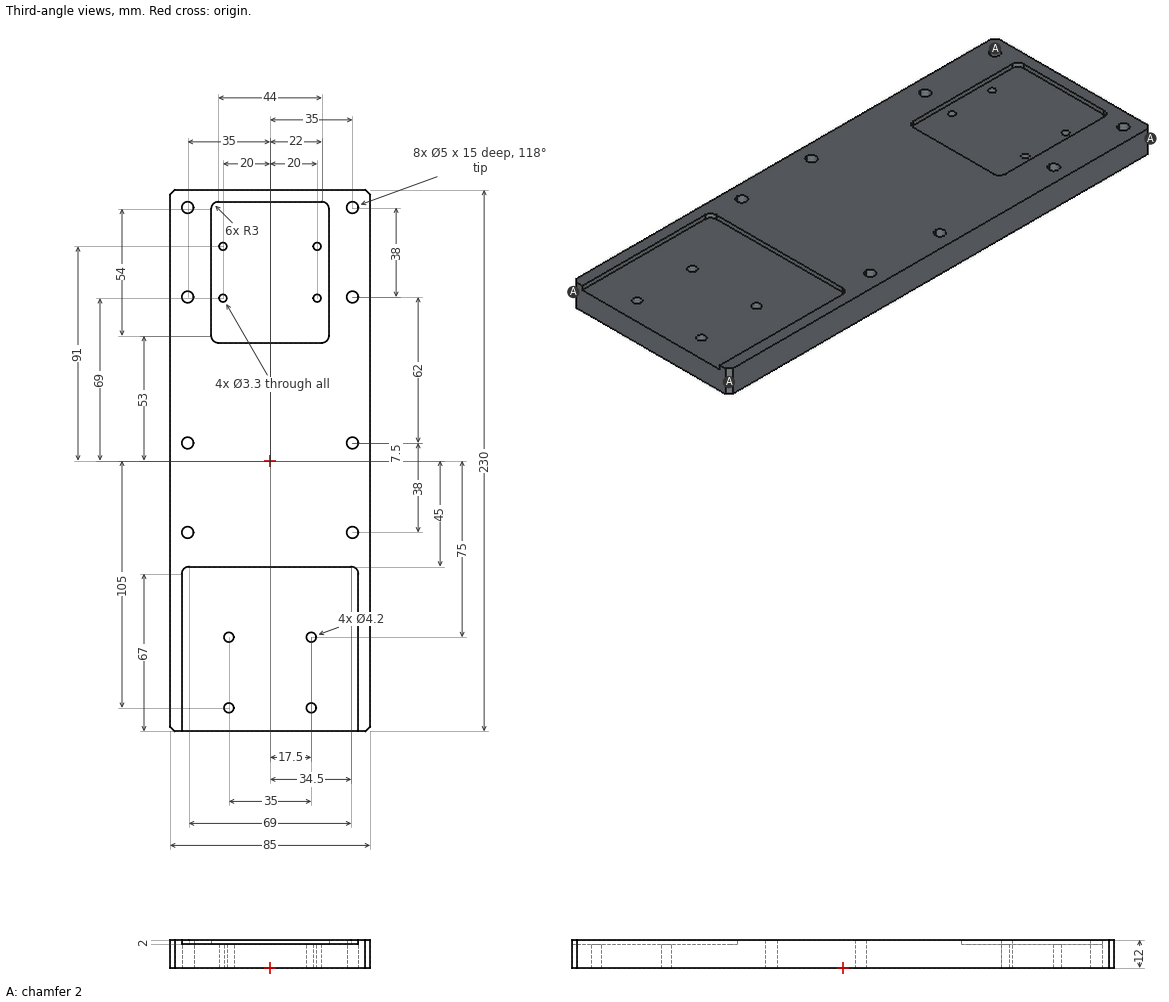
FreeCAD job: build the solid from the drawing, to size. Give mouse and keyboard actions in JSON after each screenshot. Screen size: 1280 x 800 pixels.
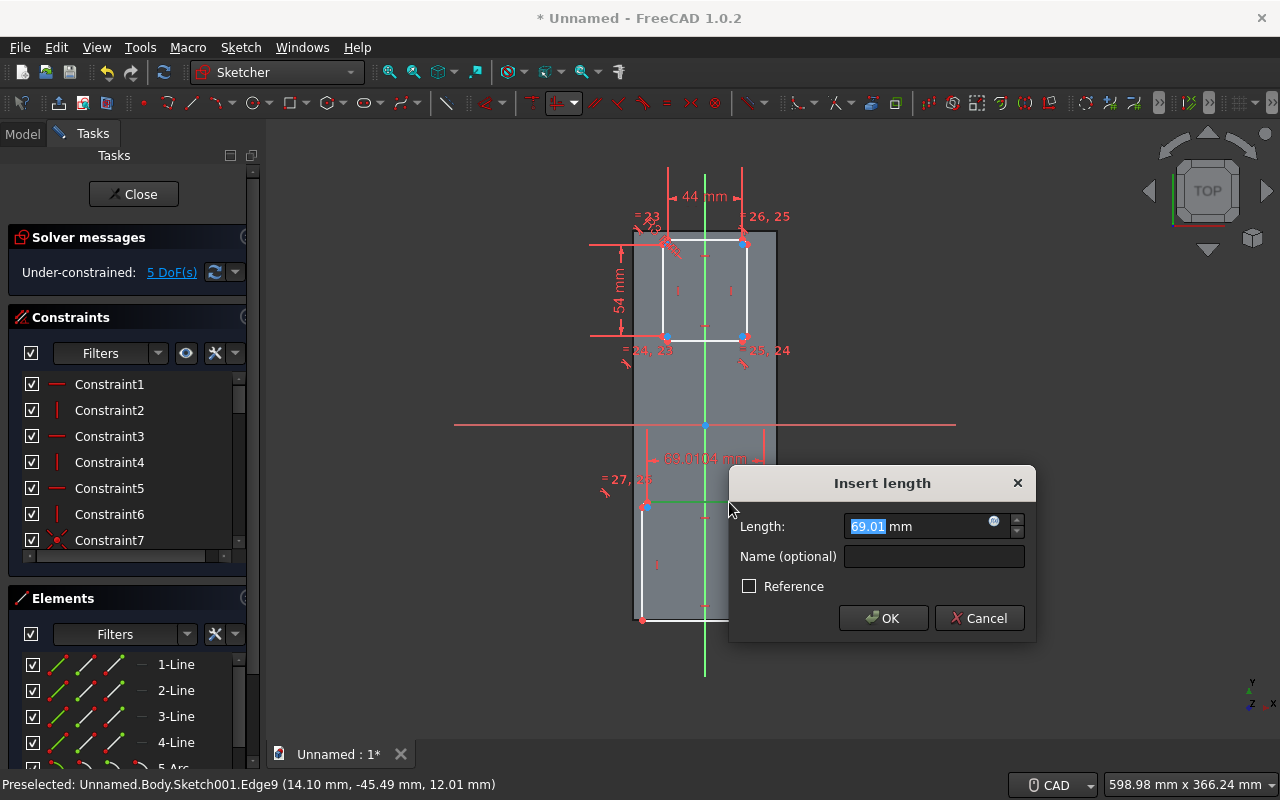
{"action": "type", "text": "69"}
{"action": "key", "text": "Return"}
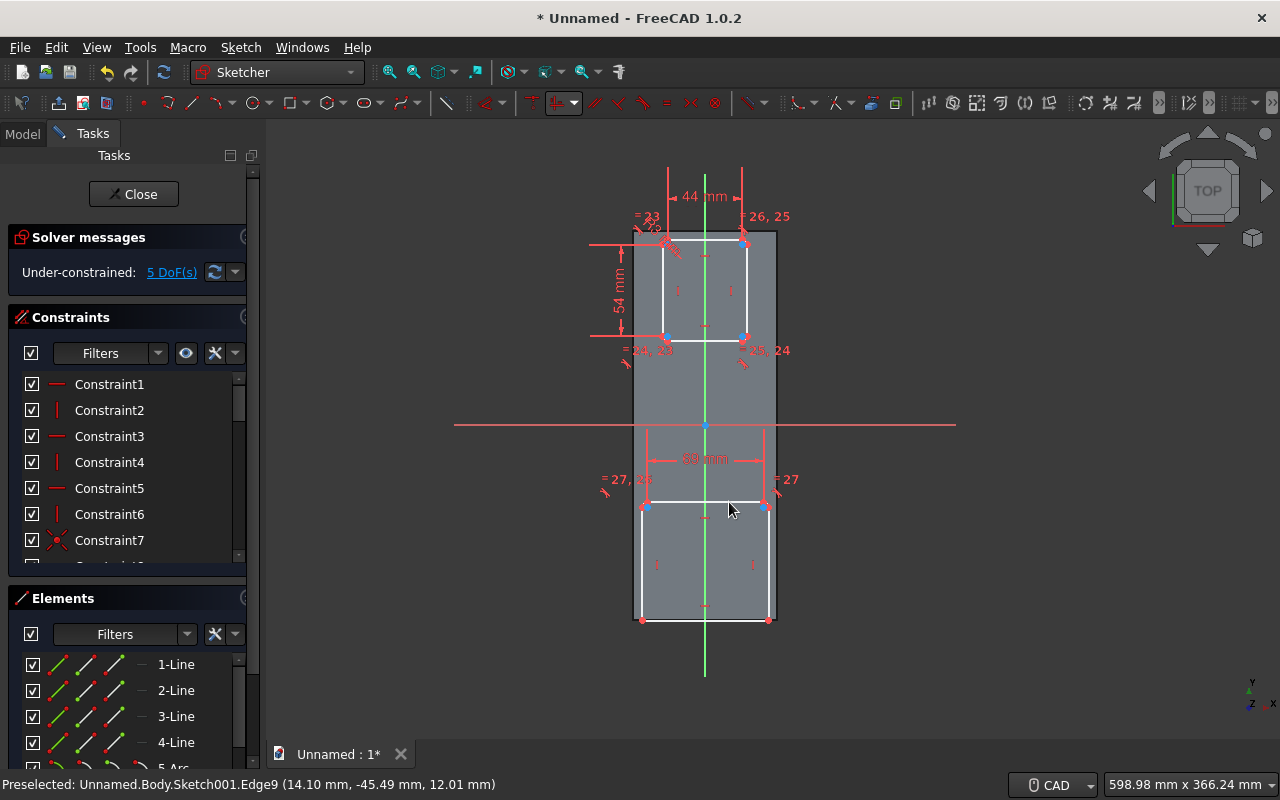
{"action": "left_click", "coordinate": [642, 541]}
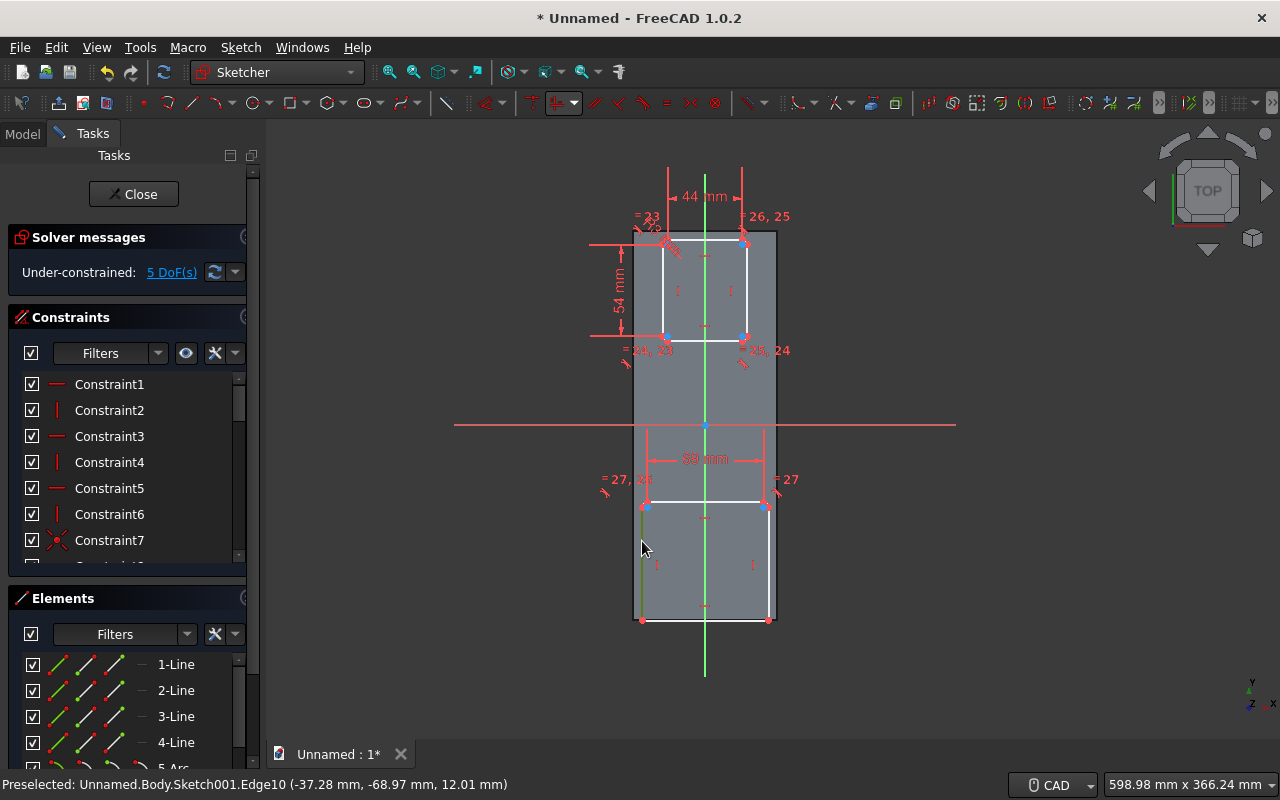
{"action": "key", "text": "i"}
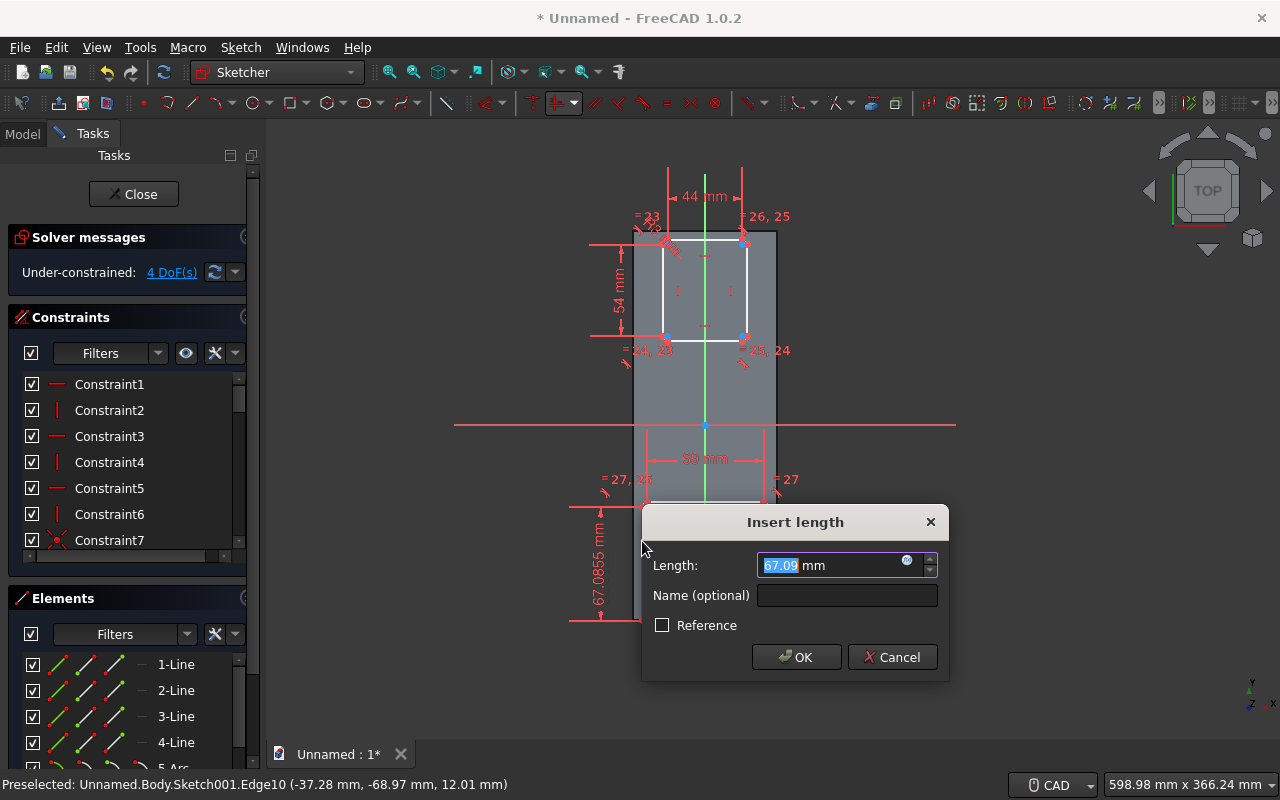
{"action": "type", "text": "67"}
{"action": "key", "text": "Return"}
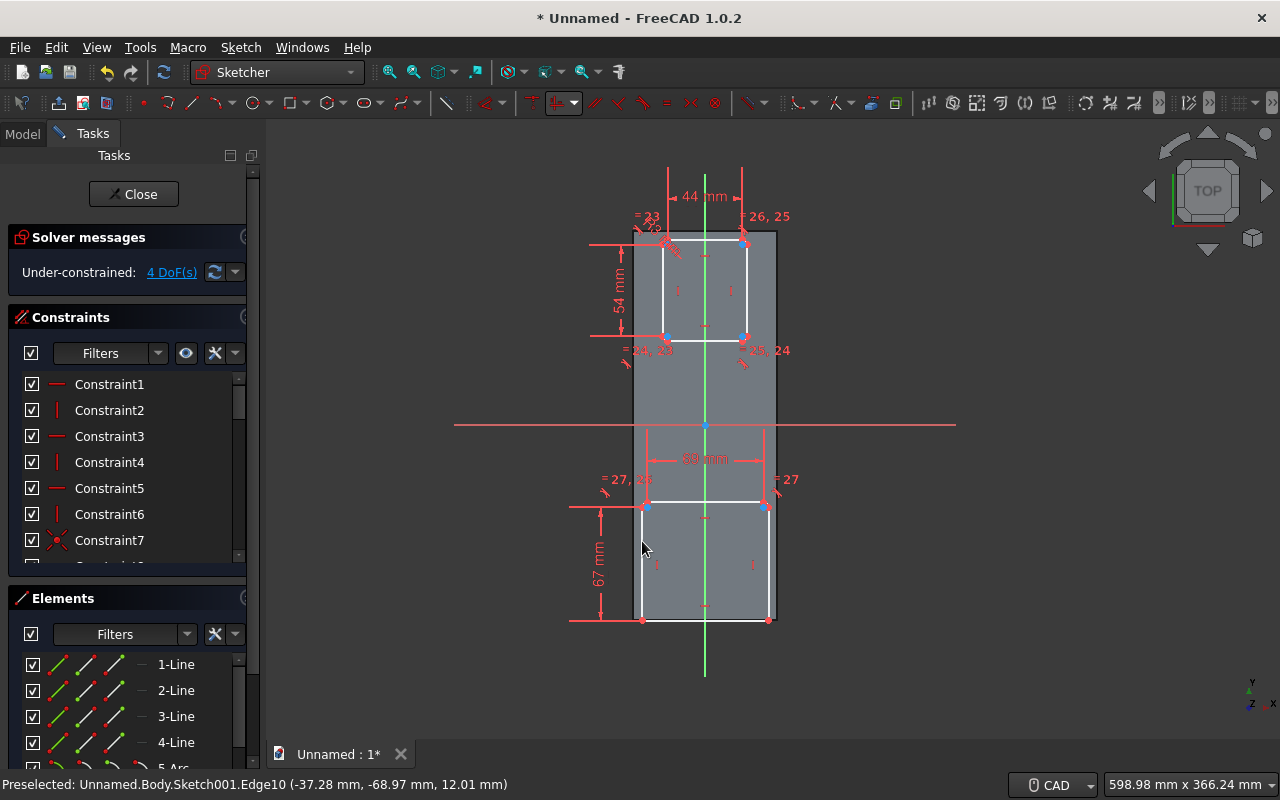
{"action": "scroll", "coordinate": [742, 240], "scroll_direction": "up", "scroll_amount": 5}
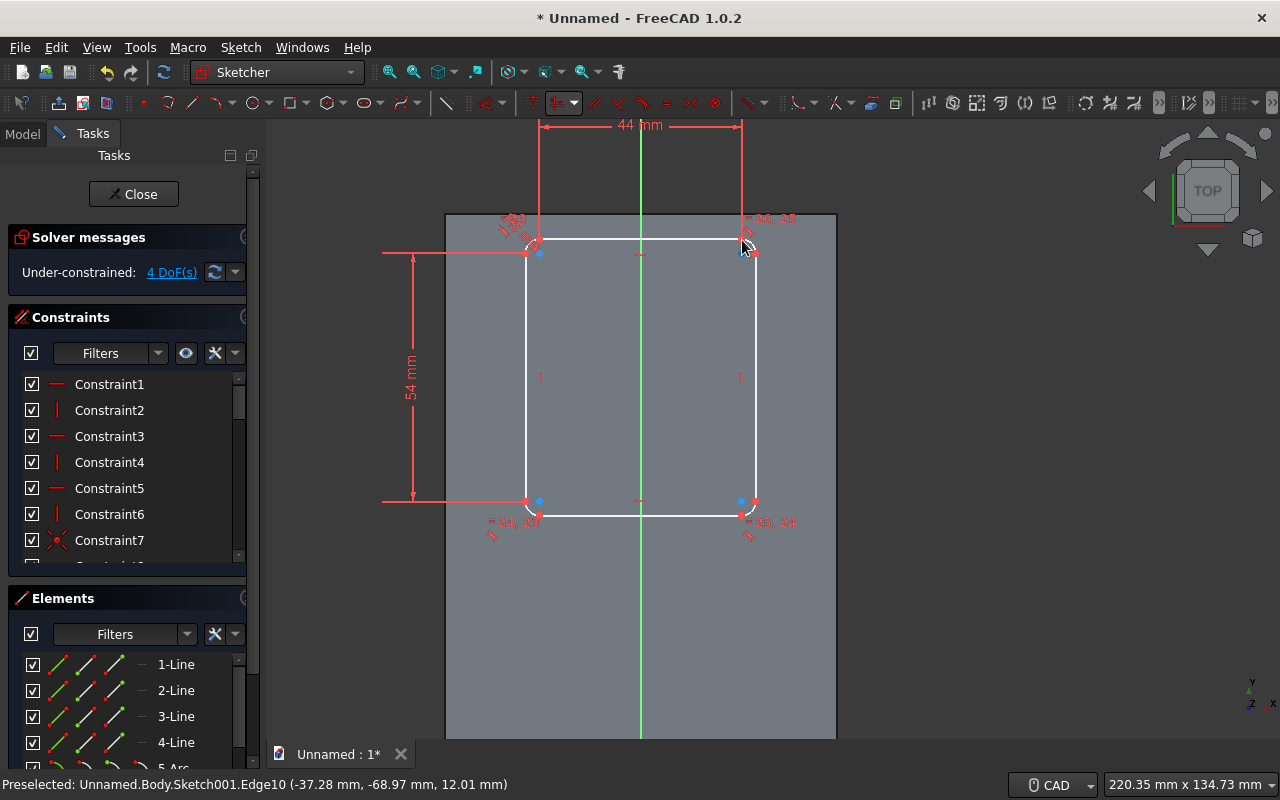
{"action": "left_click", "coordinate": [742, 239]}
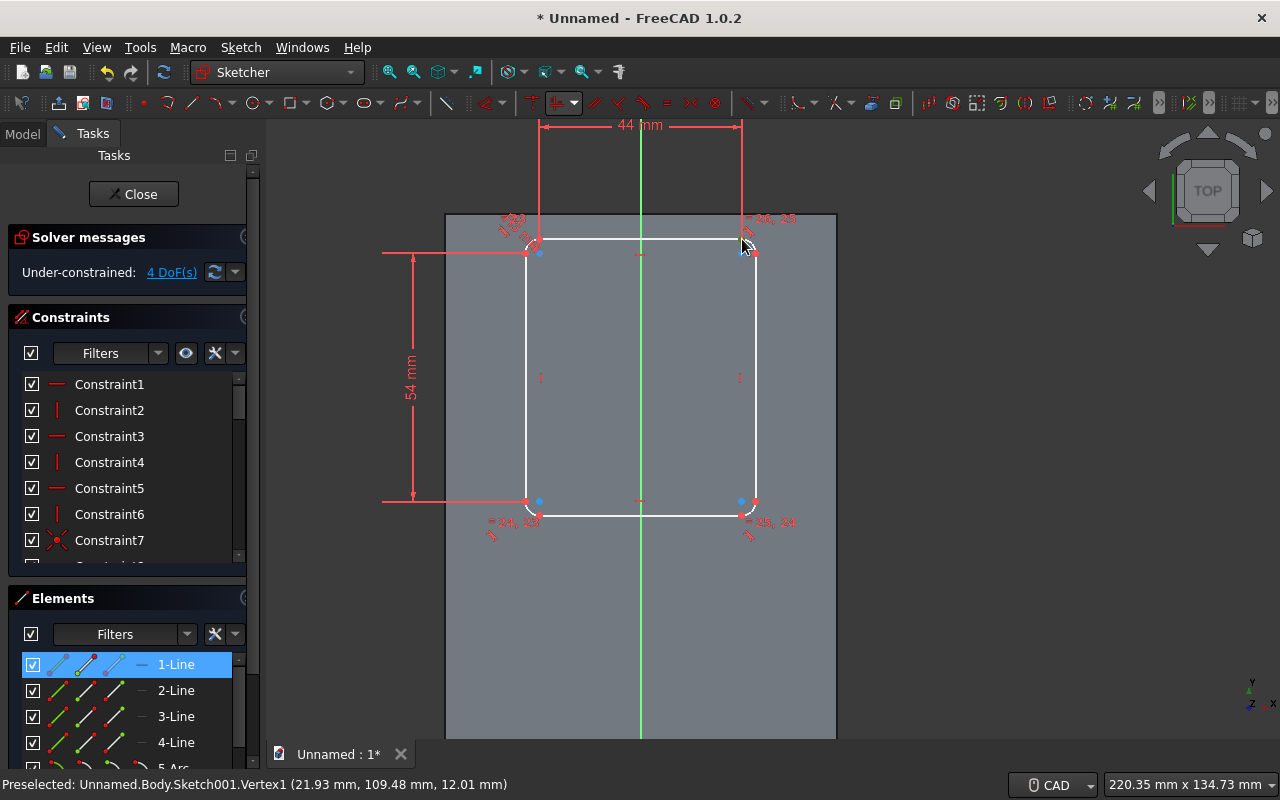
{"action": "key", "text": "l"}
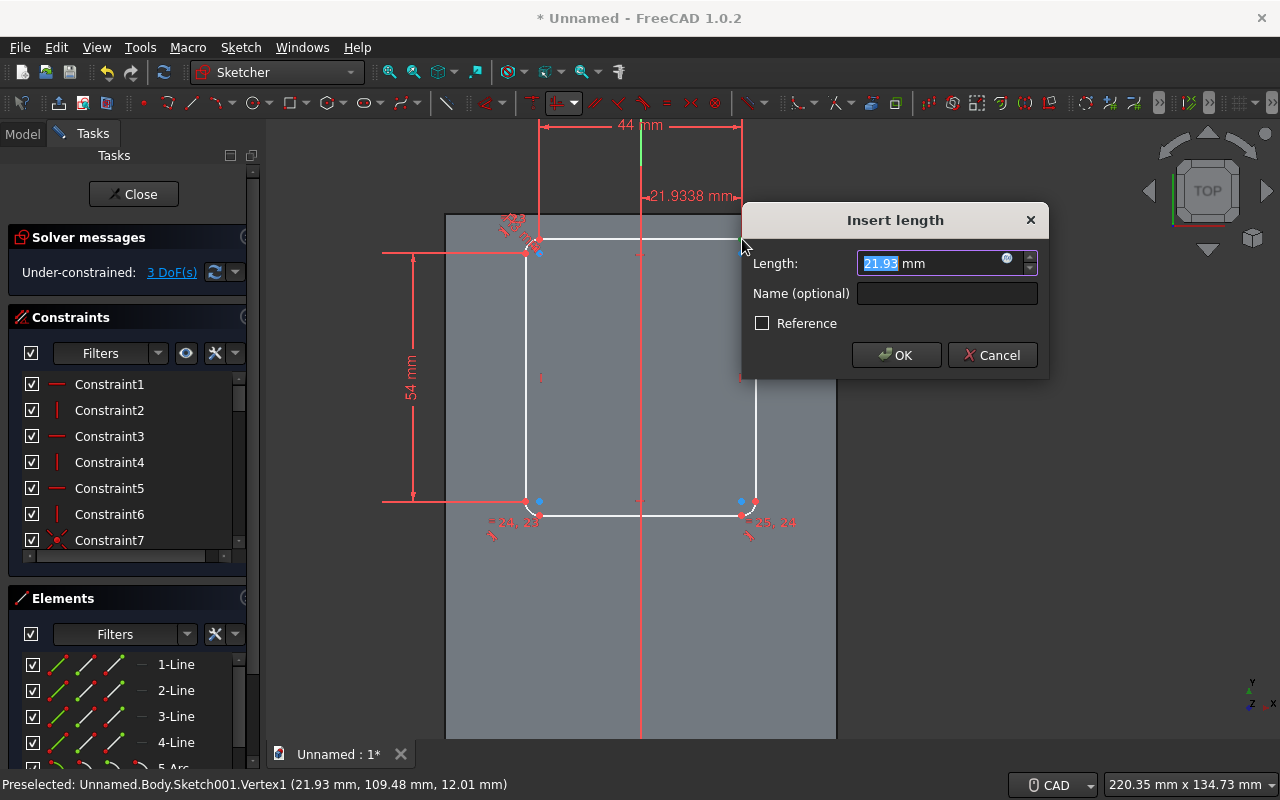
{"action": "type", "text": "22"}
{"action": "key", "text": "Return"}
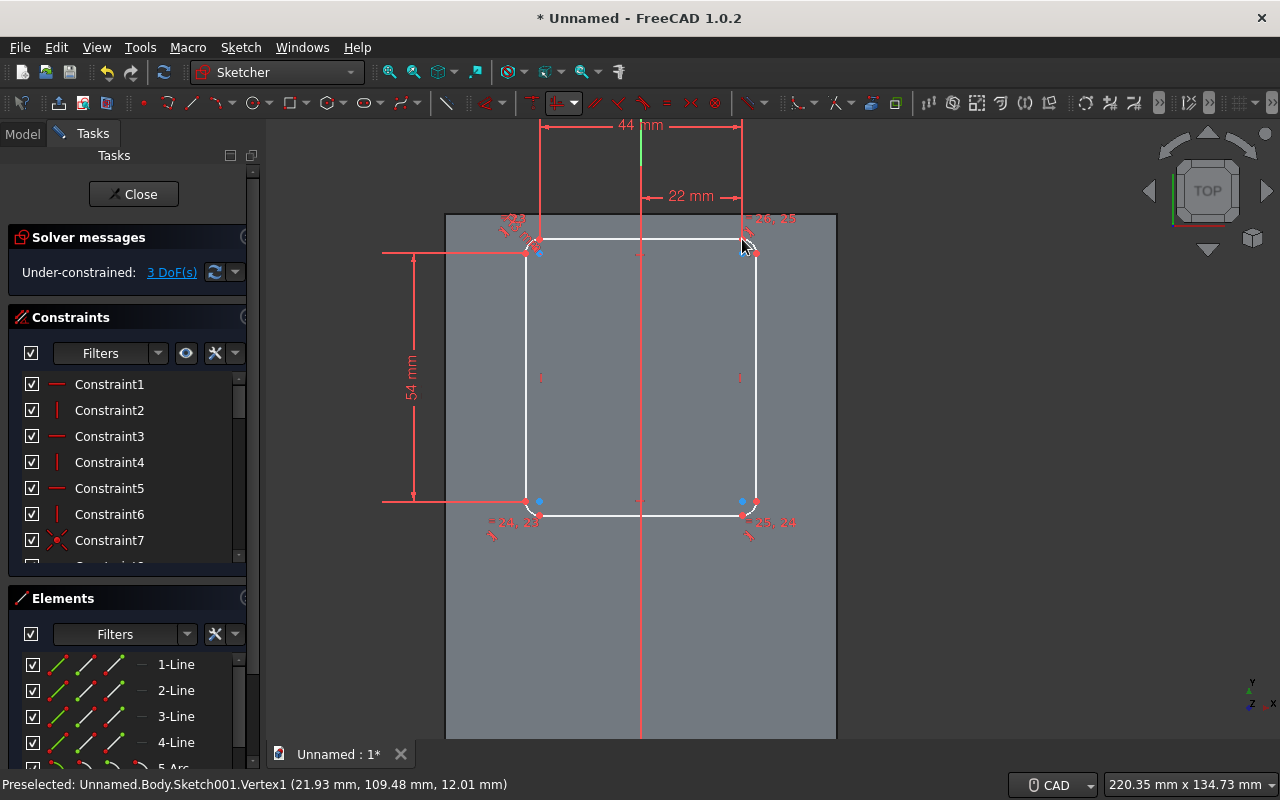
{"action": "left_click", "coordinate": [526, 502]}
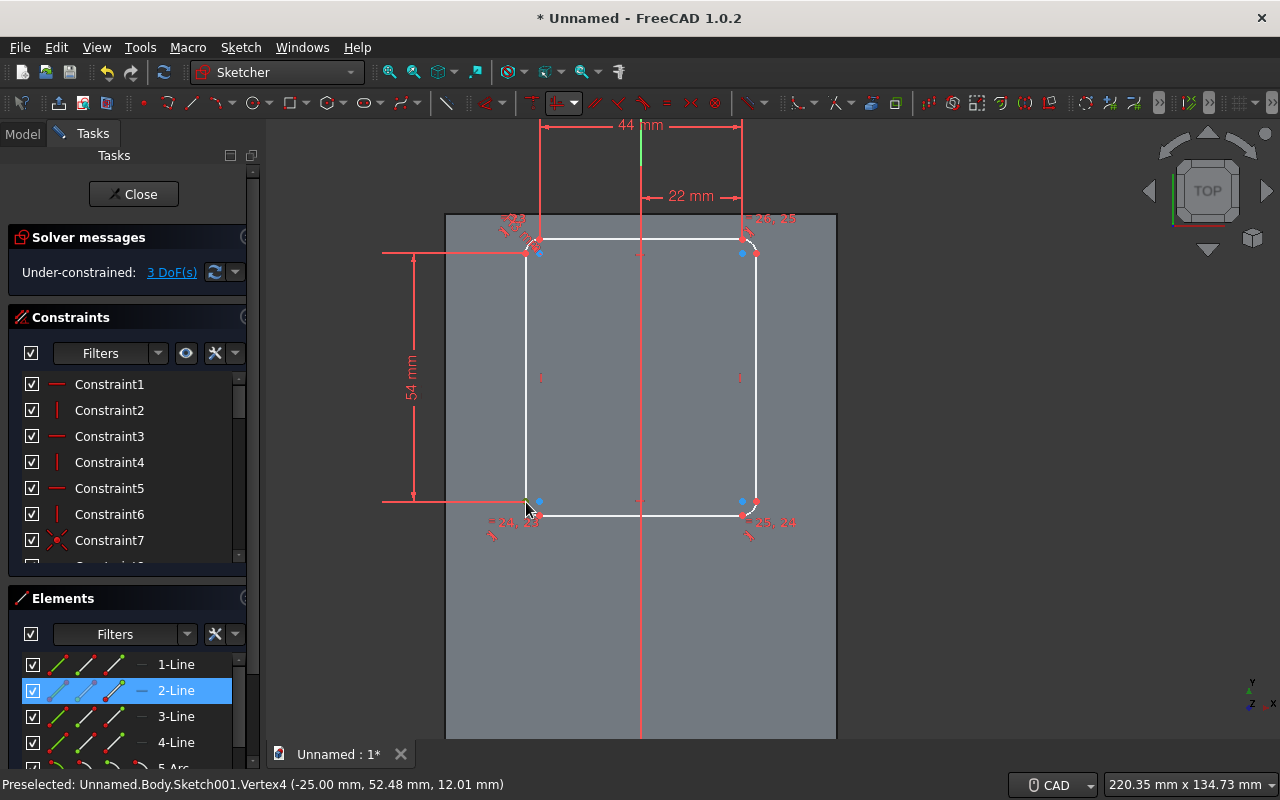
{"action": "key", "text": "i"}